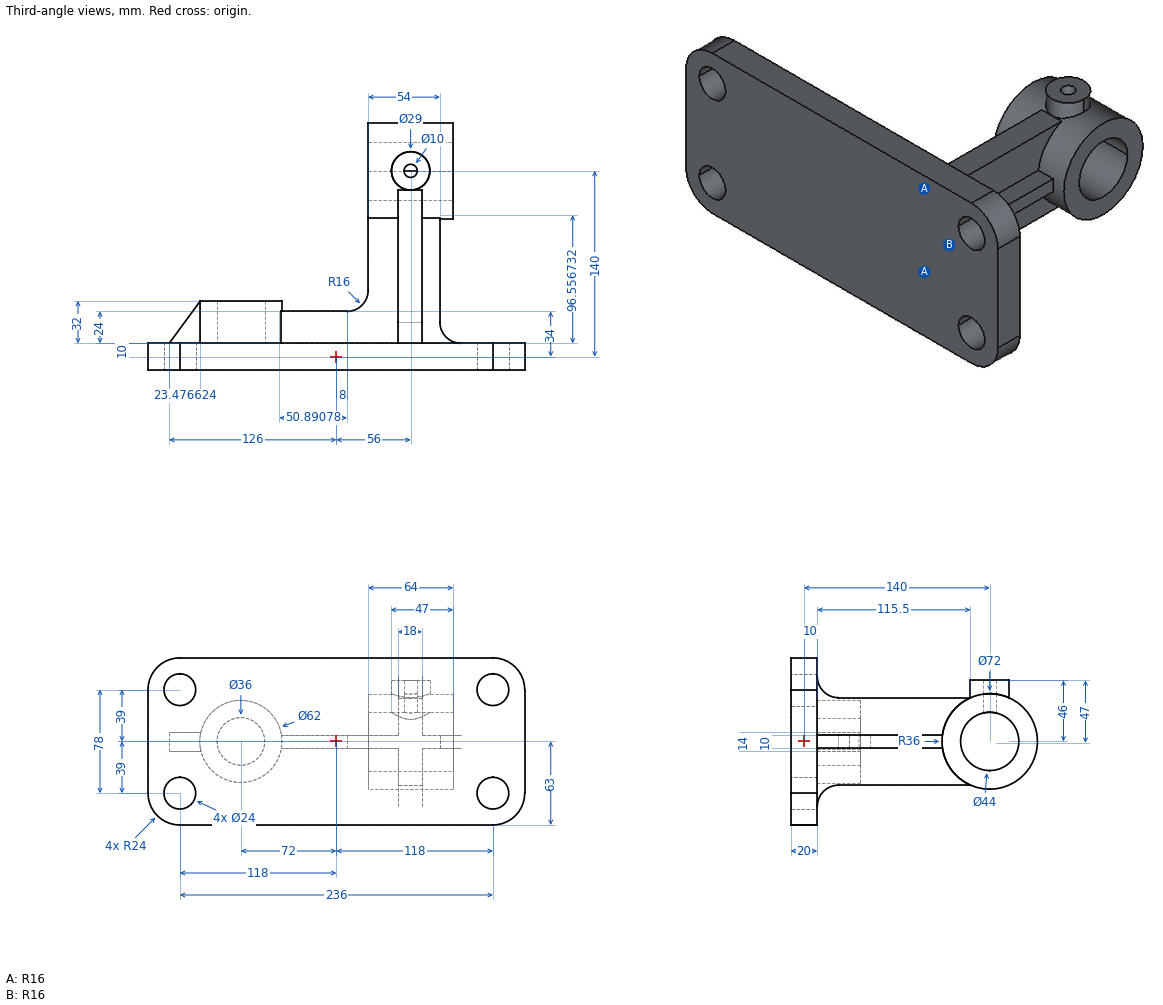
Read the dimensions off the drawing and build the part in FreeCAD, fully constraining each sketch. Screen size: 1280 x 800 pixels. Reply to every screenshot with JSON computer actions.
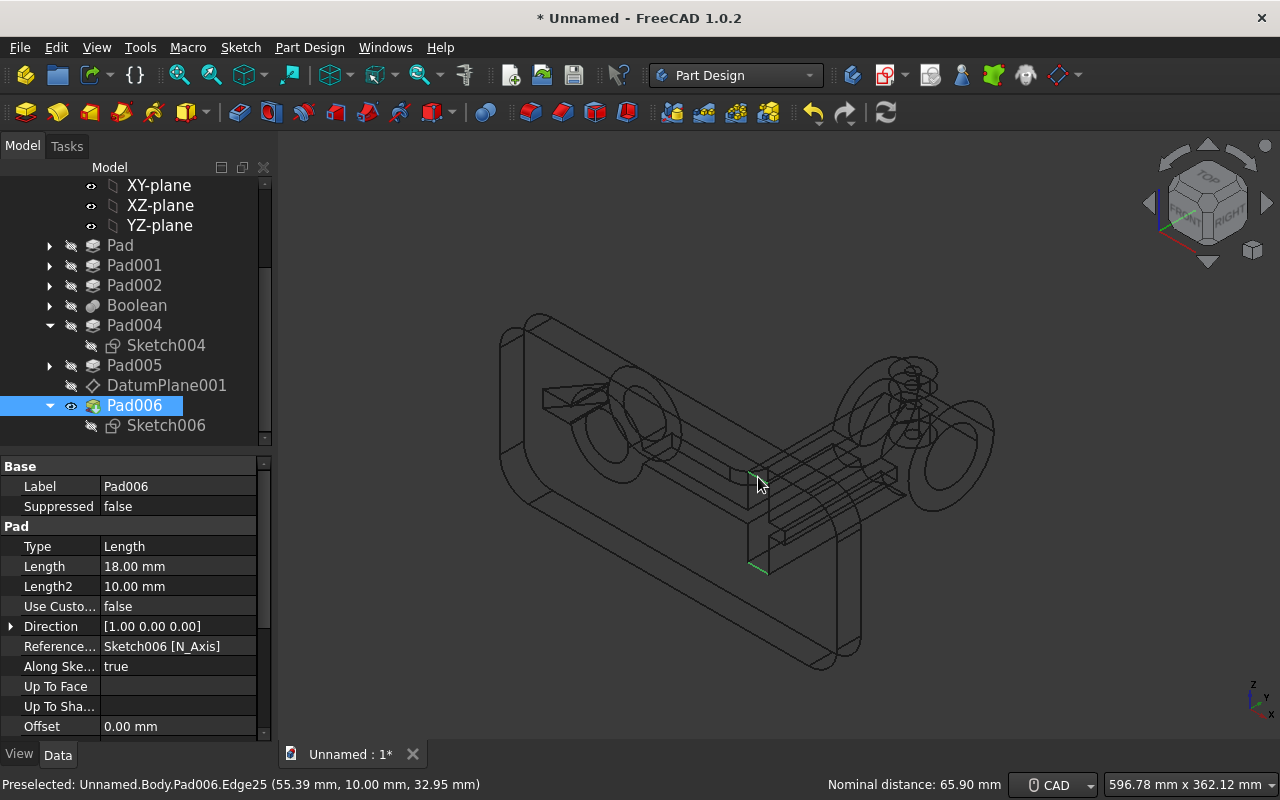
{"action": "key", "text": "v 1"}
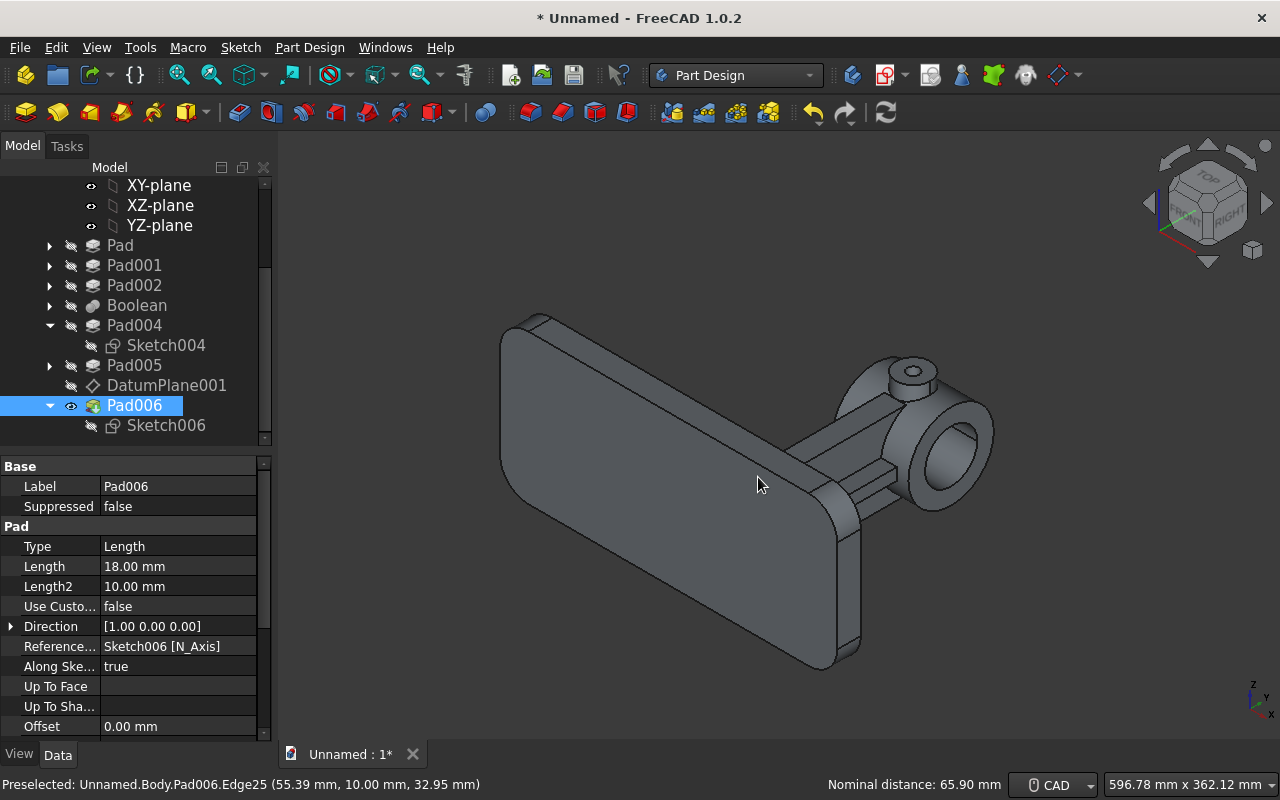
{"action": "left_click", "coordinate": [532, 112]}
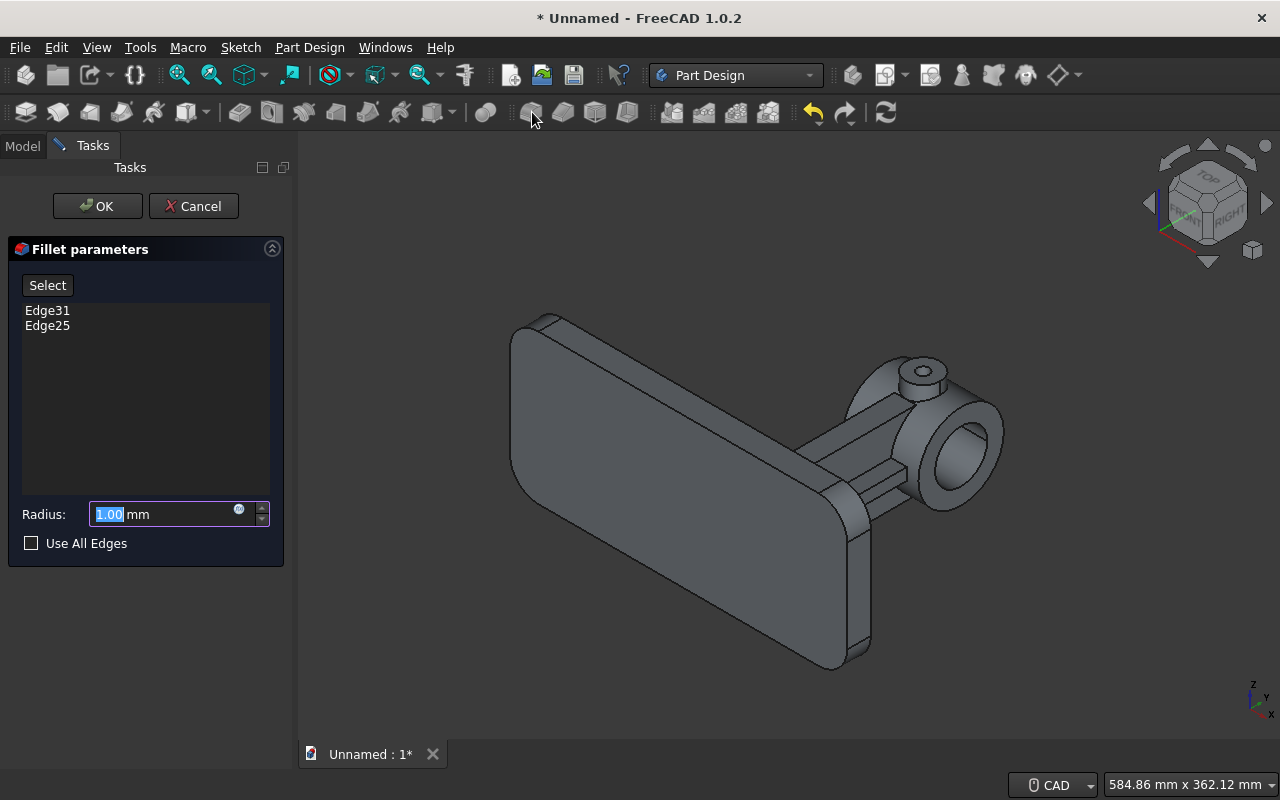
{"action": "type", "text": "16"}
{"action": "key", "text": "Tab"}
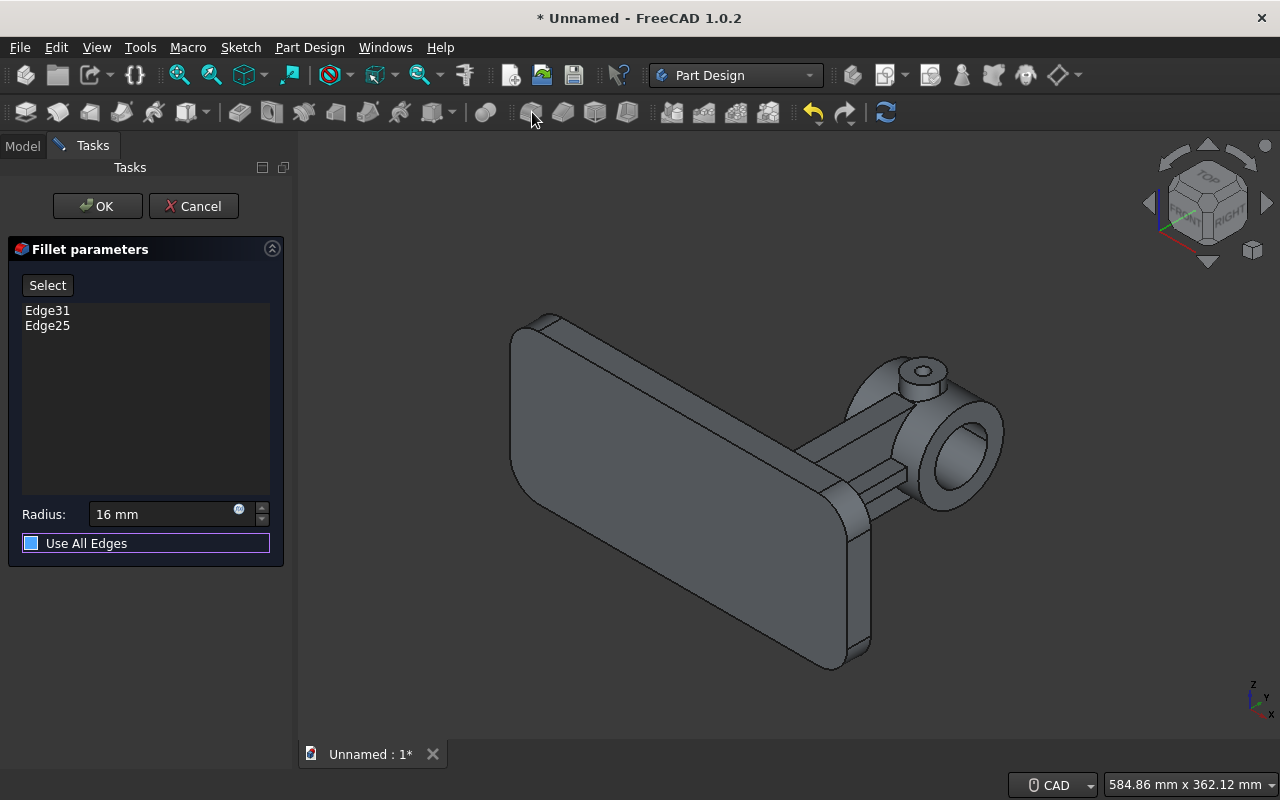
{"action": "left_click", "coordinate": [98, 206]}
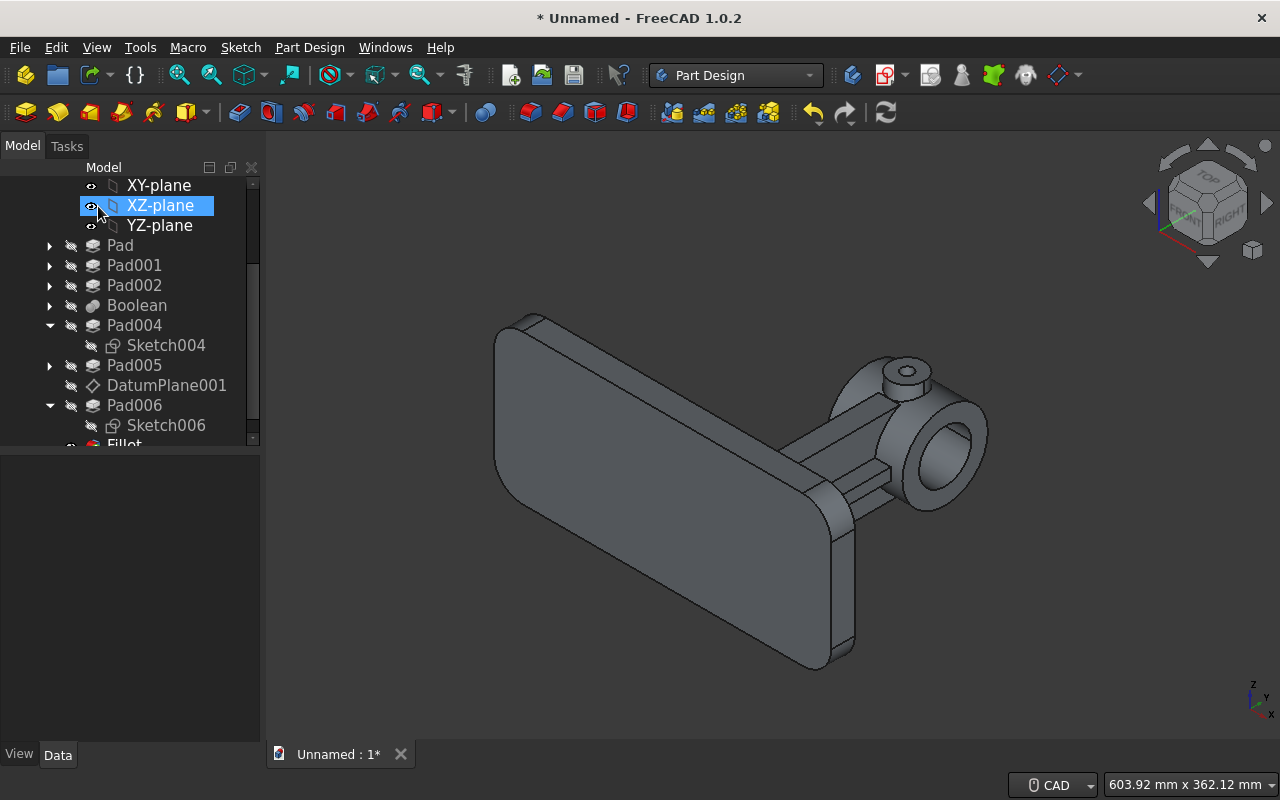
{"action": "key", "text": "4"}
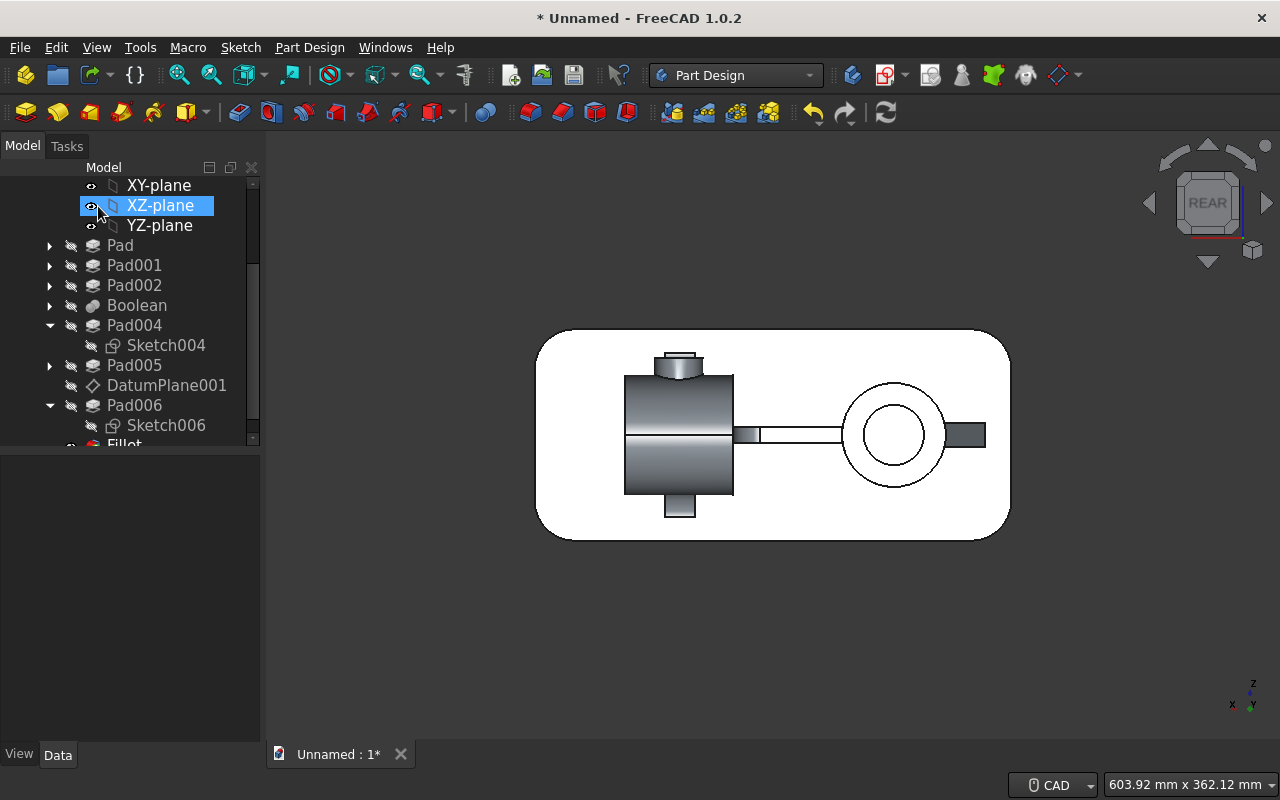
{"action": "left_click", "coordinate": [773, 374]}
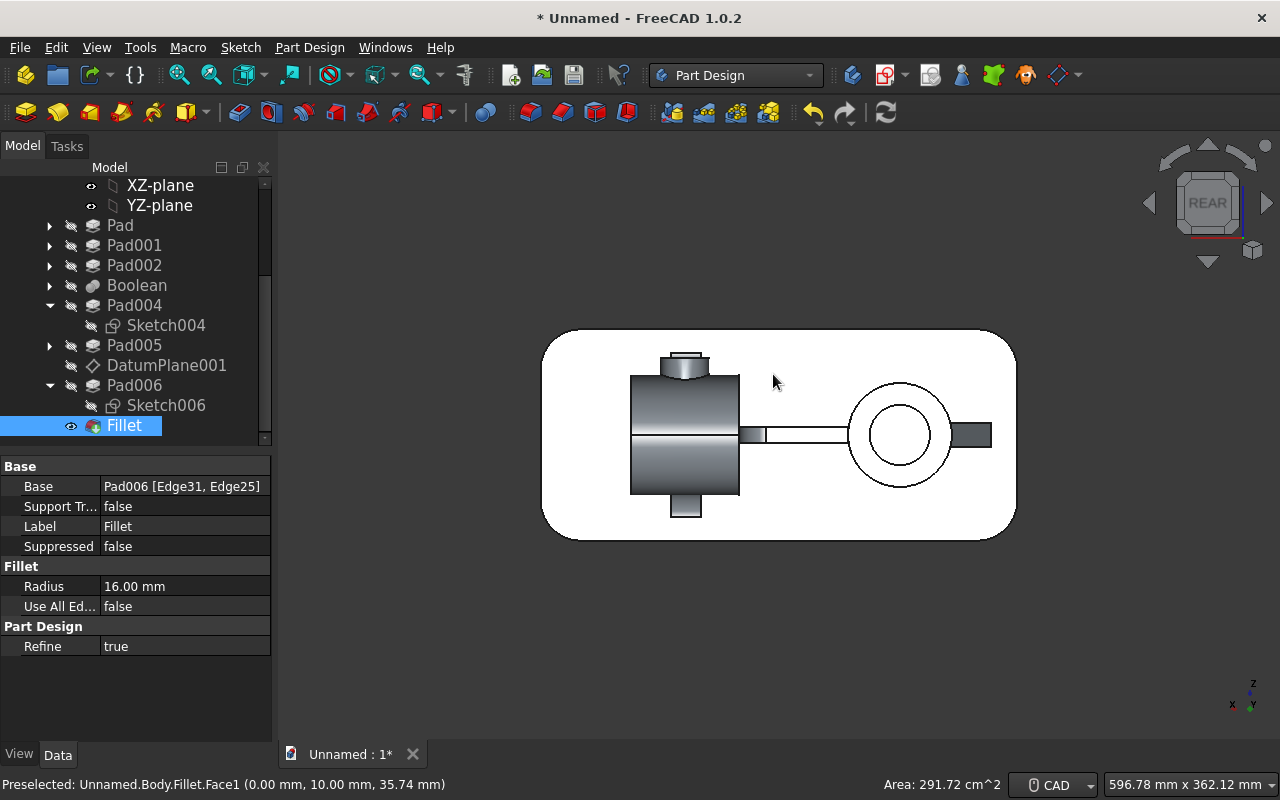
{"action": "left_click", "coordinate": [886, 76]}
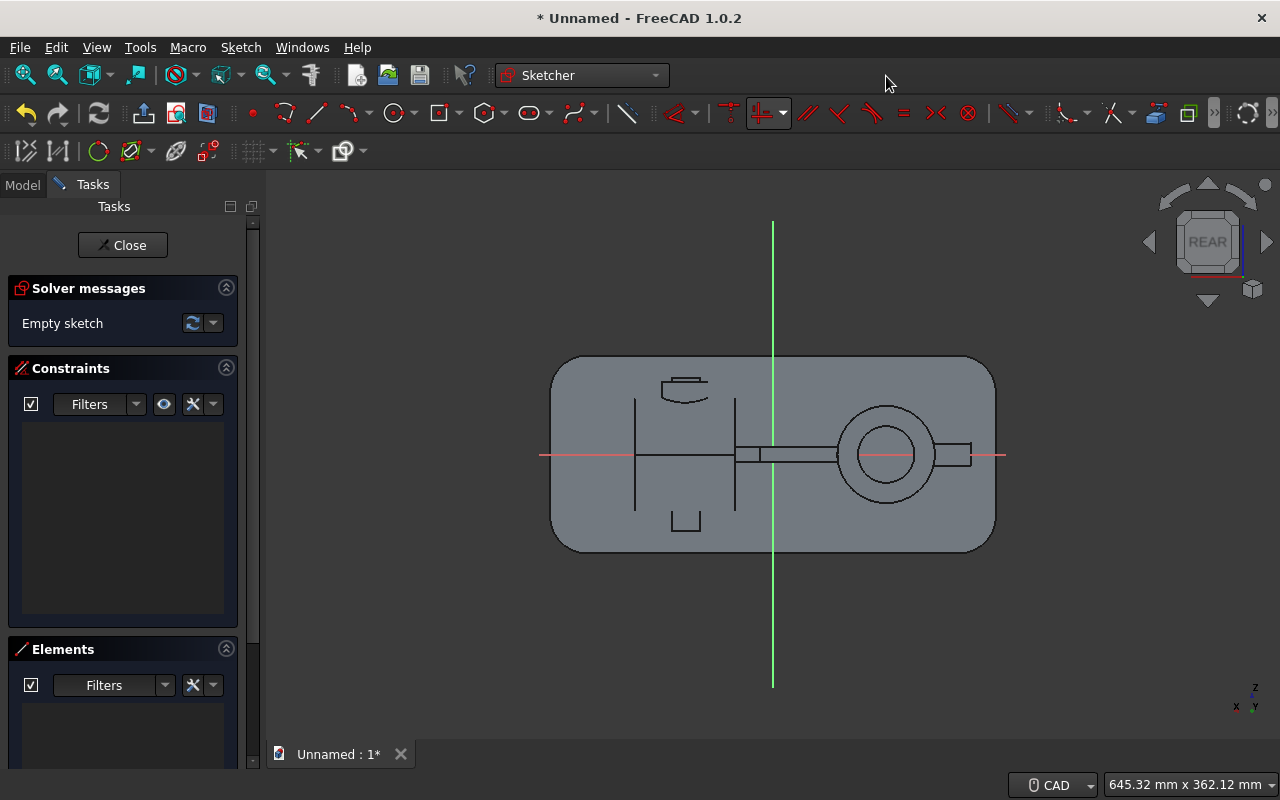
{"action": "scroll", "coordinate": [912, 454], "scroll_direction": "up", "scroll_amount": 2}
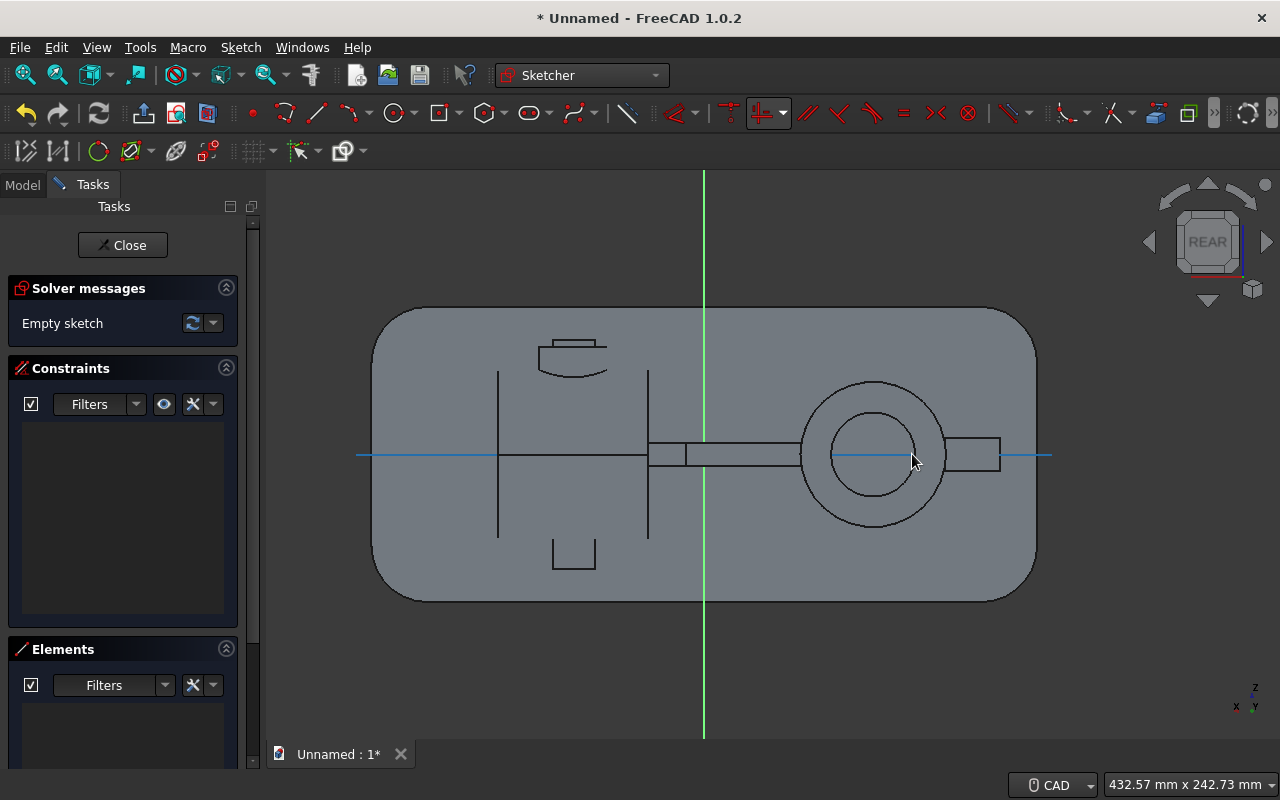
{"action": "left_click", "coordinate": [394, 114]}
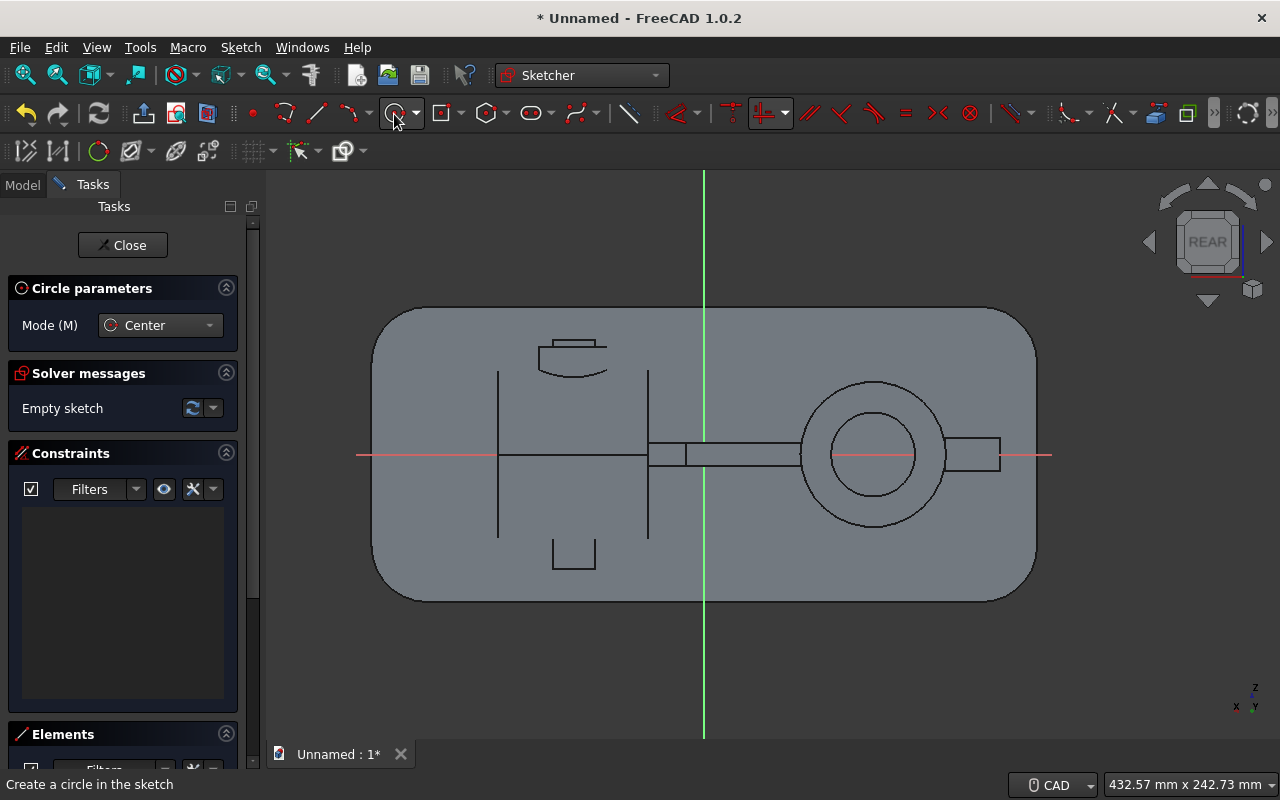
{"action": "left_click", "coordinate": [981, 546]}
{"action": "mouse_move", "coordinate": [1001, 526]}